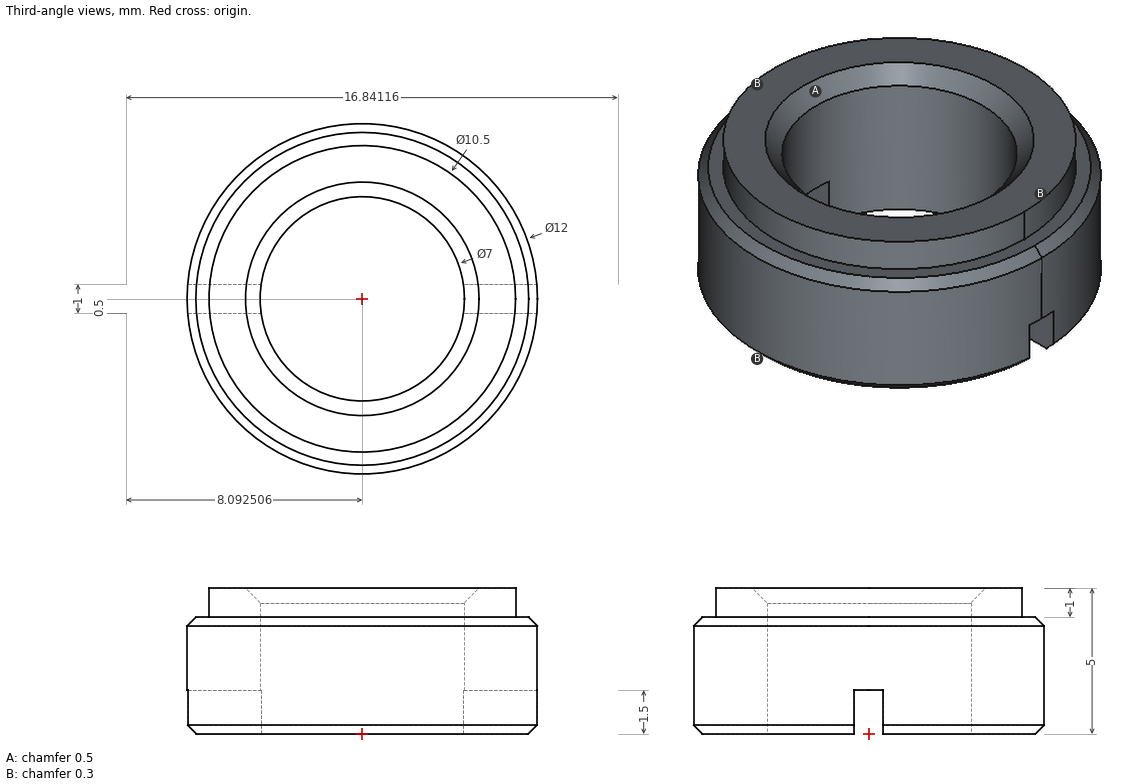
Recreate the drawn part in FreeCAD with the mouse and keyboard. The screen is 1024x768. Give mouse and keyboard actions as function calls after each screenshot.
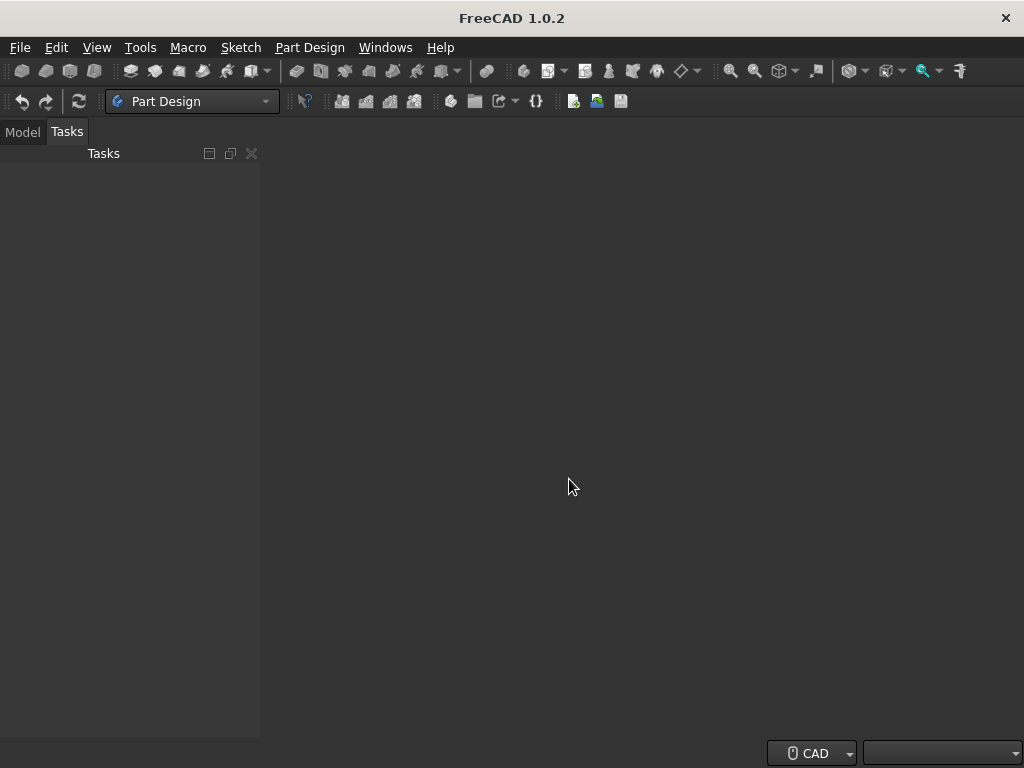
click(574, 102)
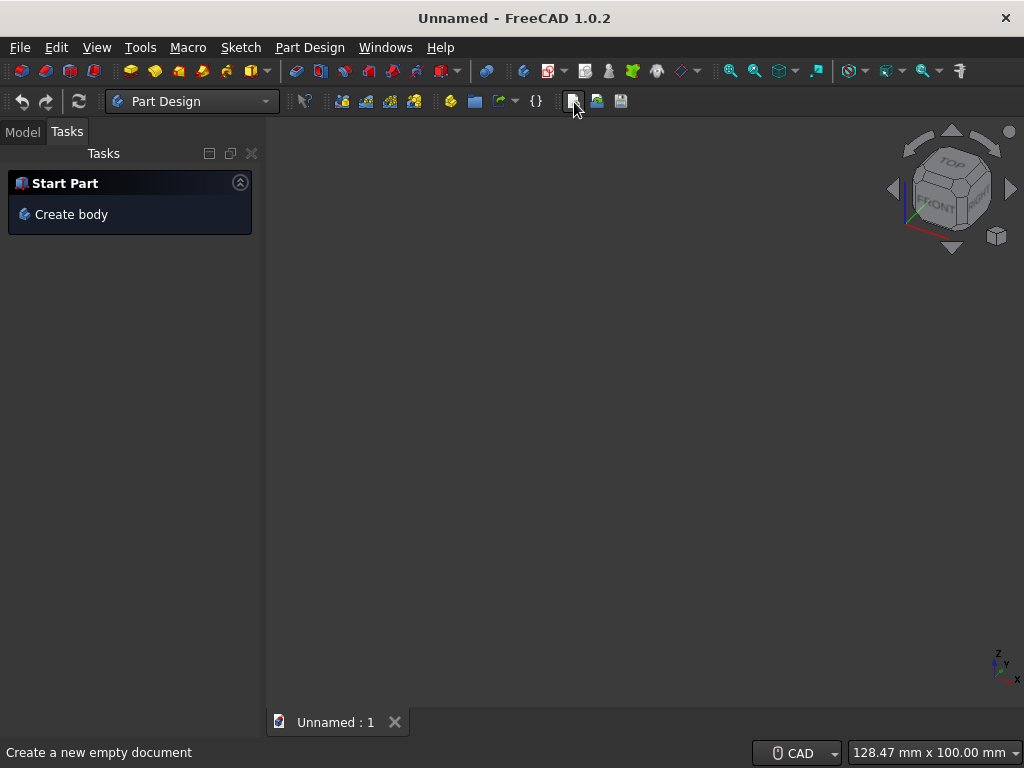
click(548, 72)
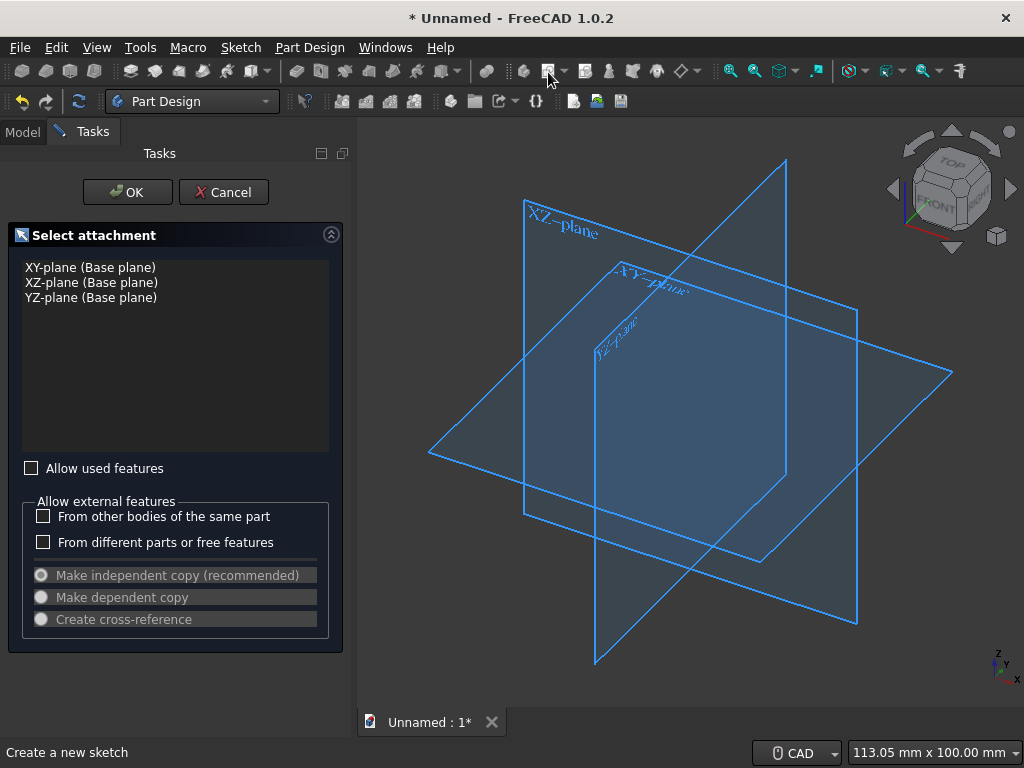
click(82, 268)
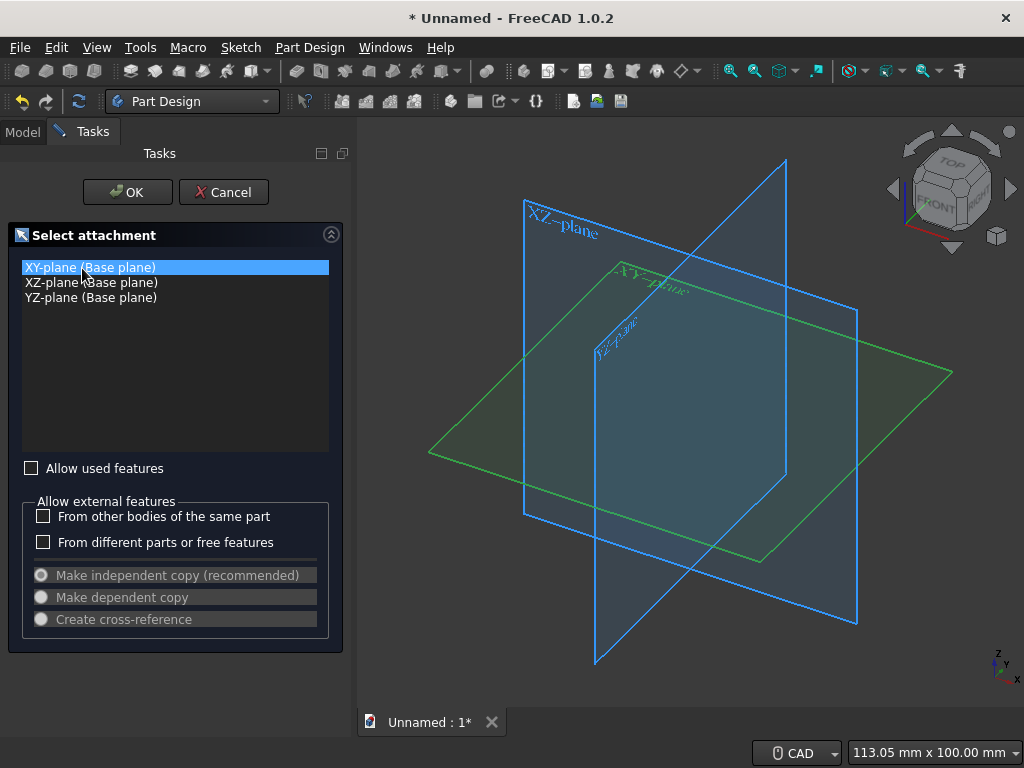
click(128, 192)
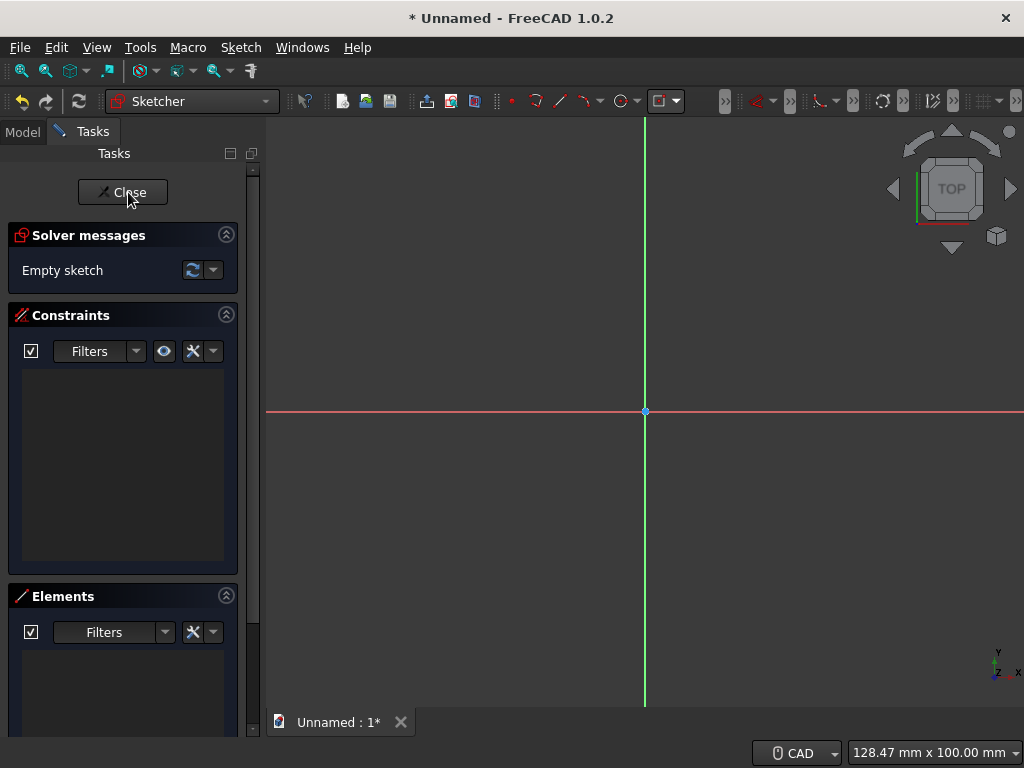
scroll(662, 412, up, 8)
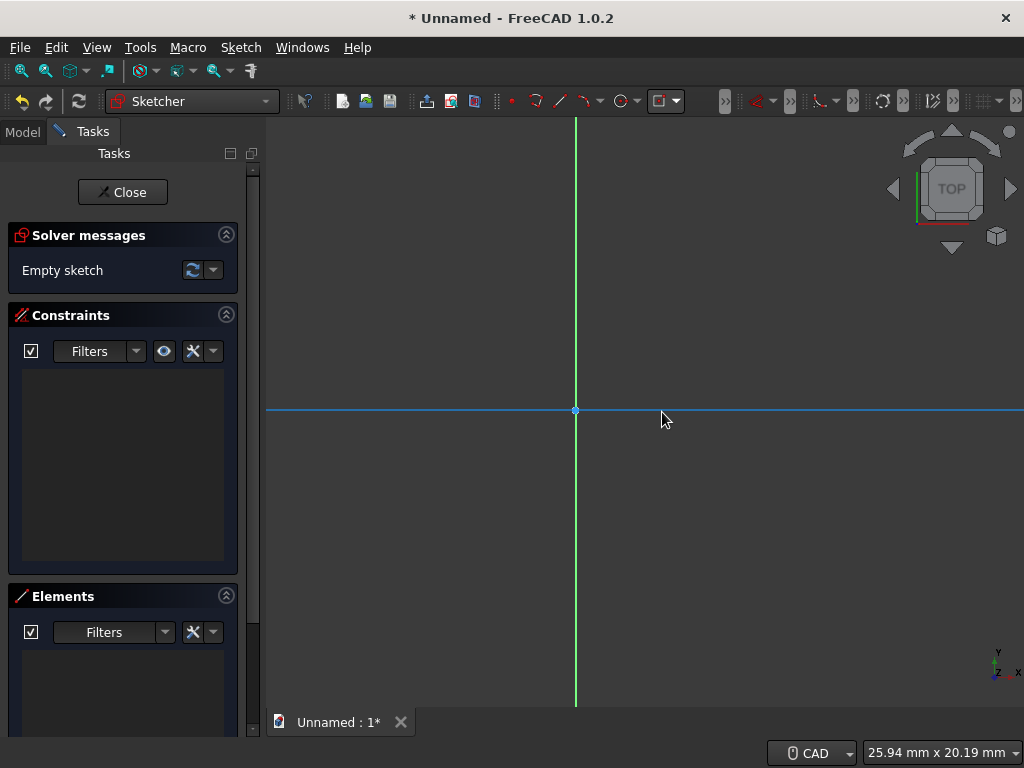
click(622, 102)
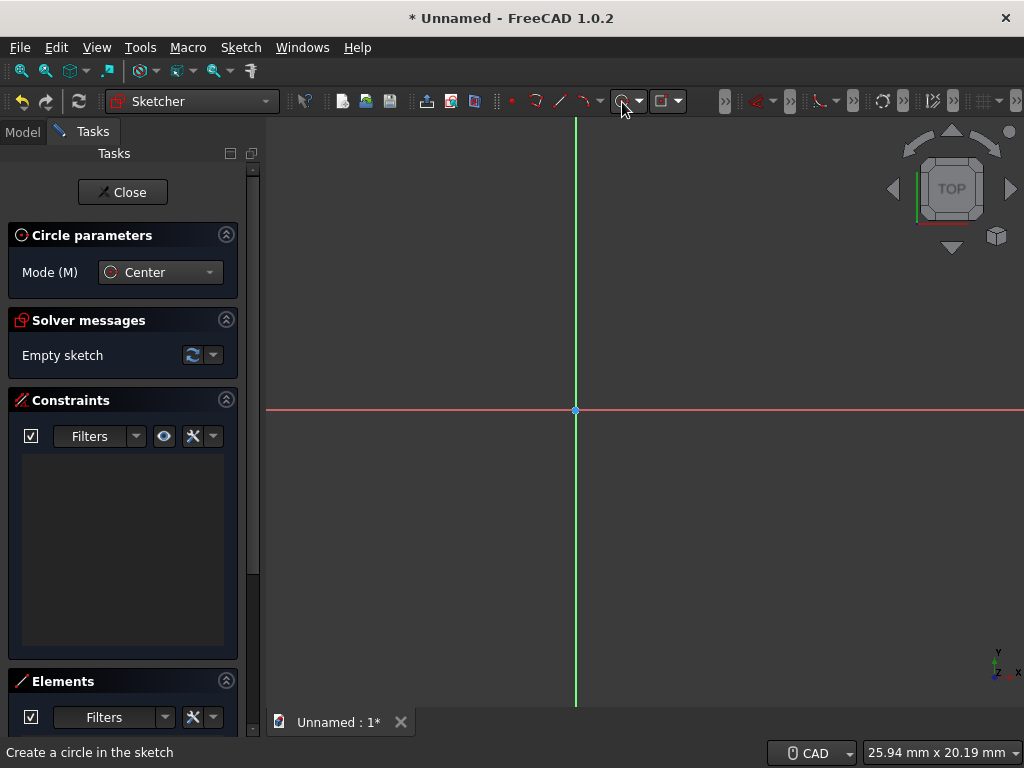
click(576, 410)
move(700, 286)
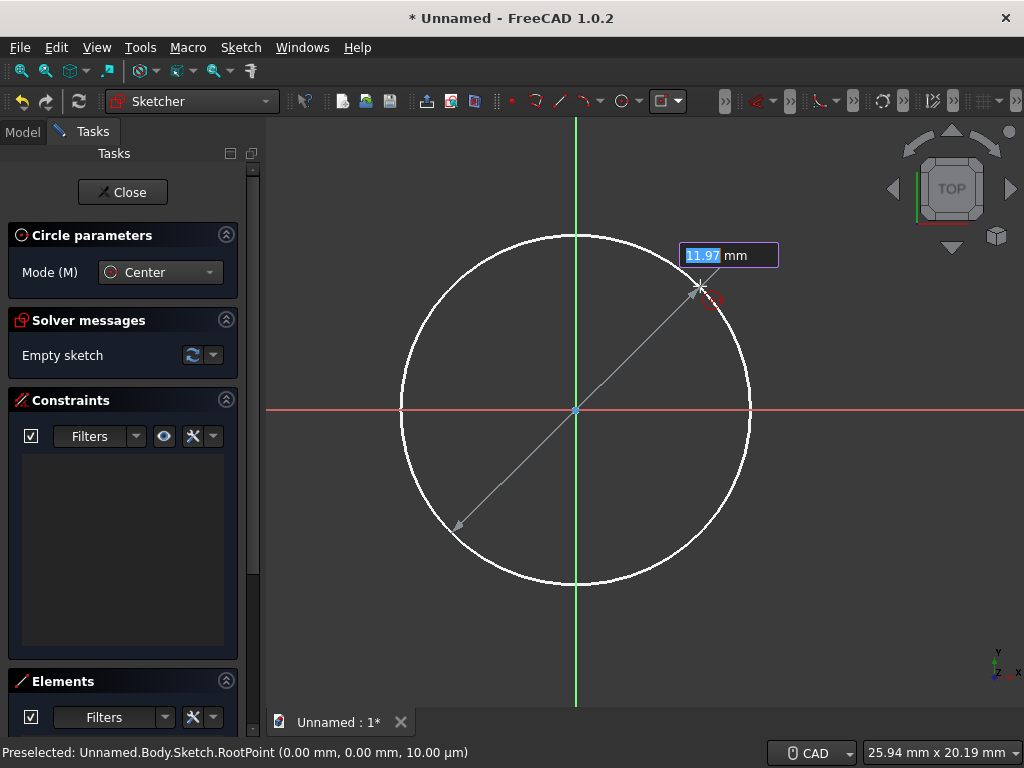
text(12)
key(Return)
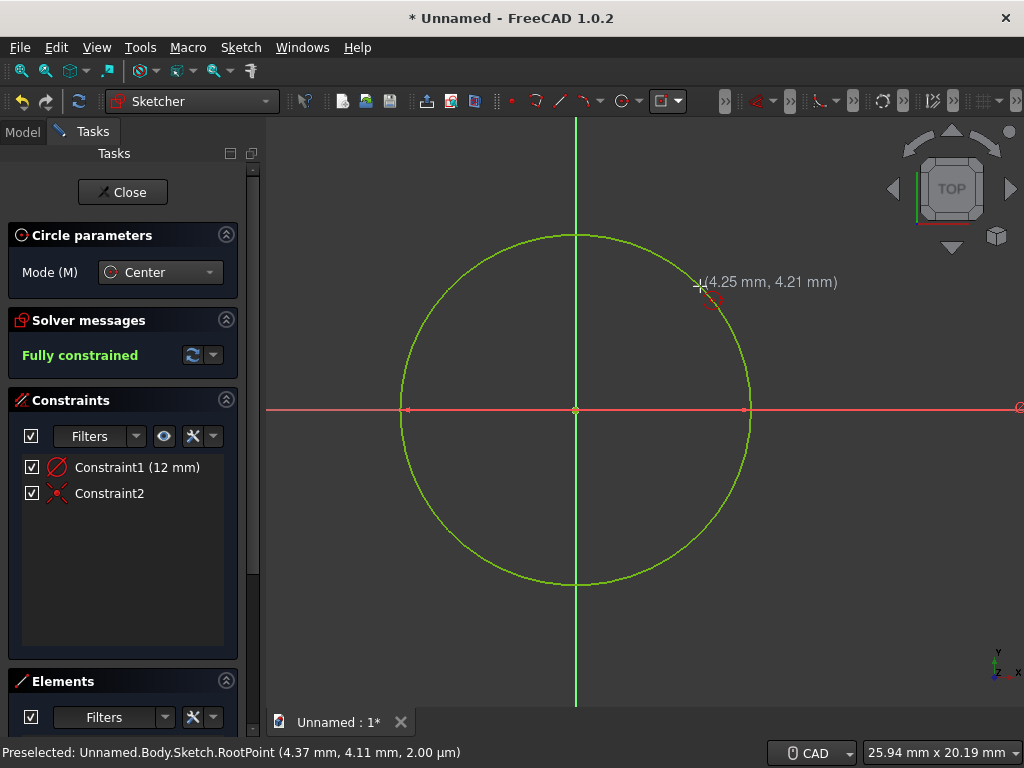
click(576, 410)
move(648, 338)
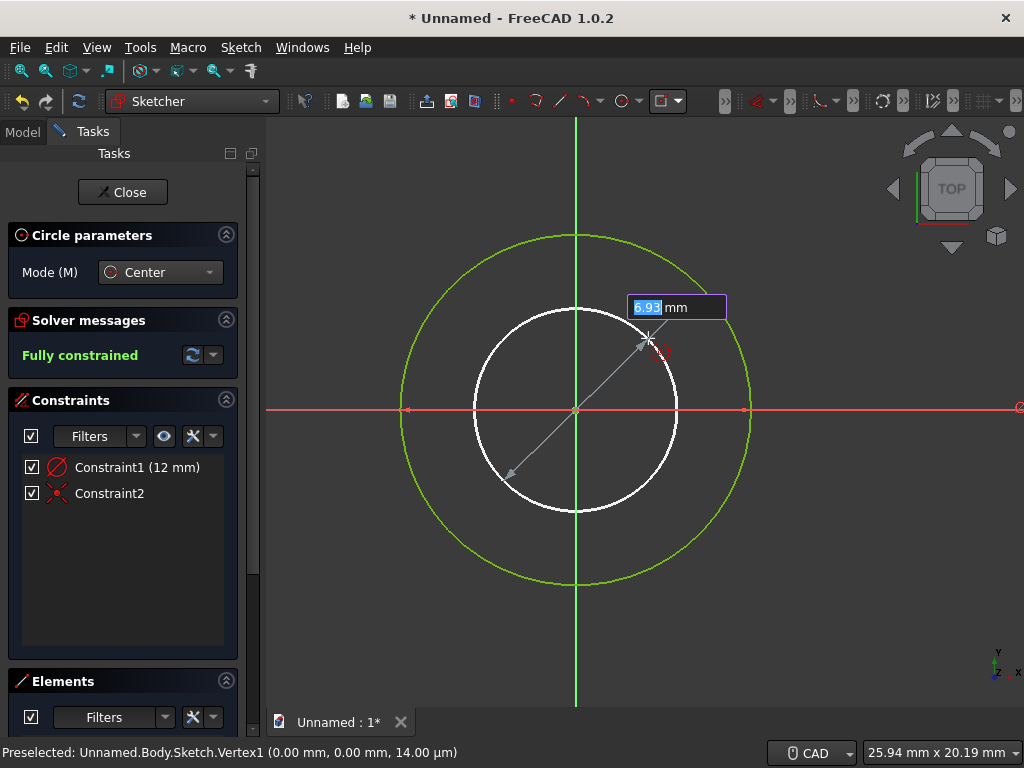
text(7)
key(Return)
key(Escape)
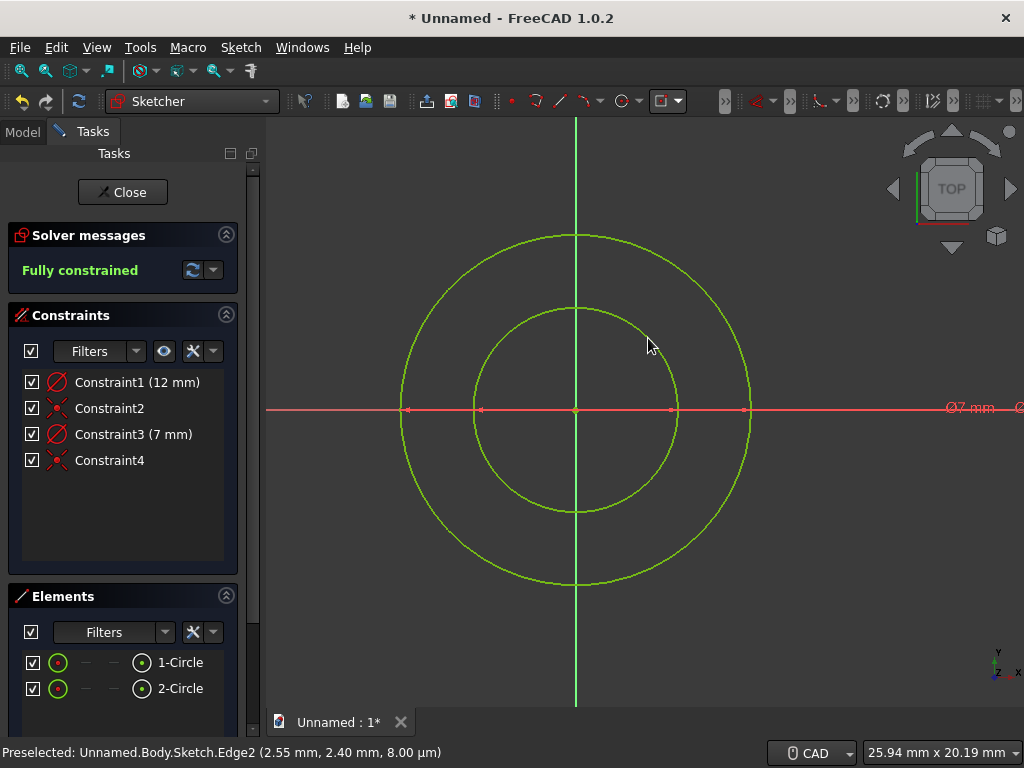
click(123, 192)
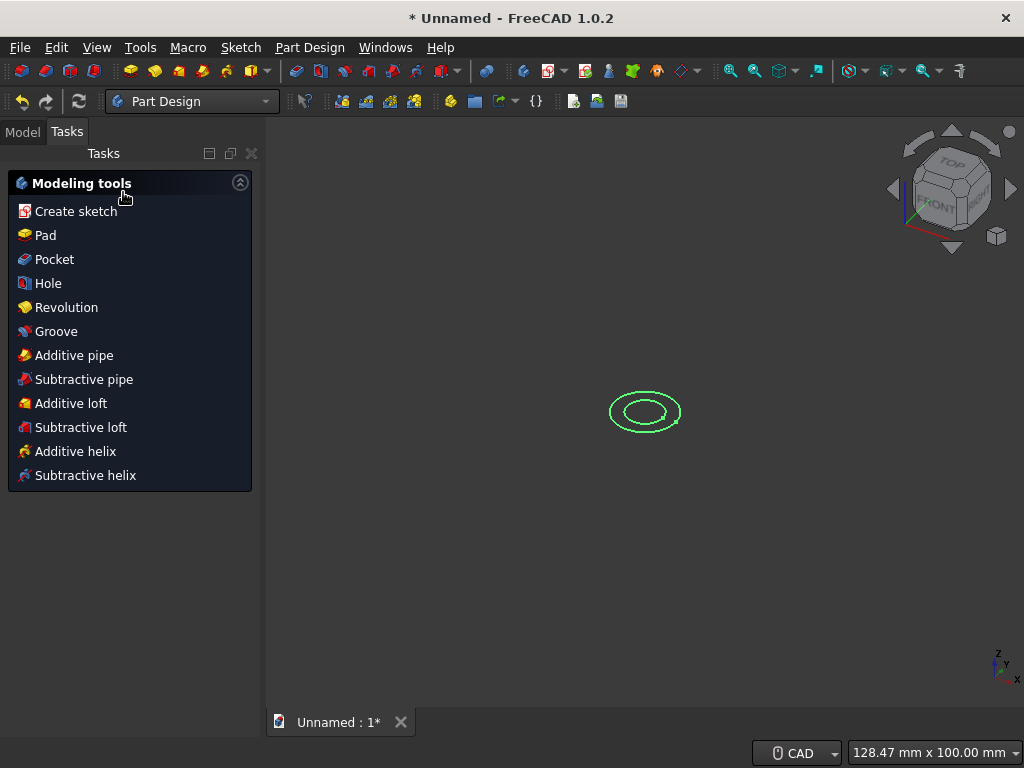
click(132, 72)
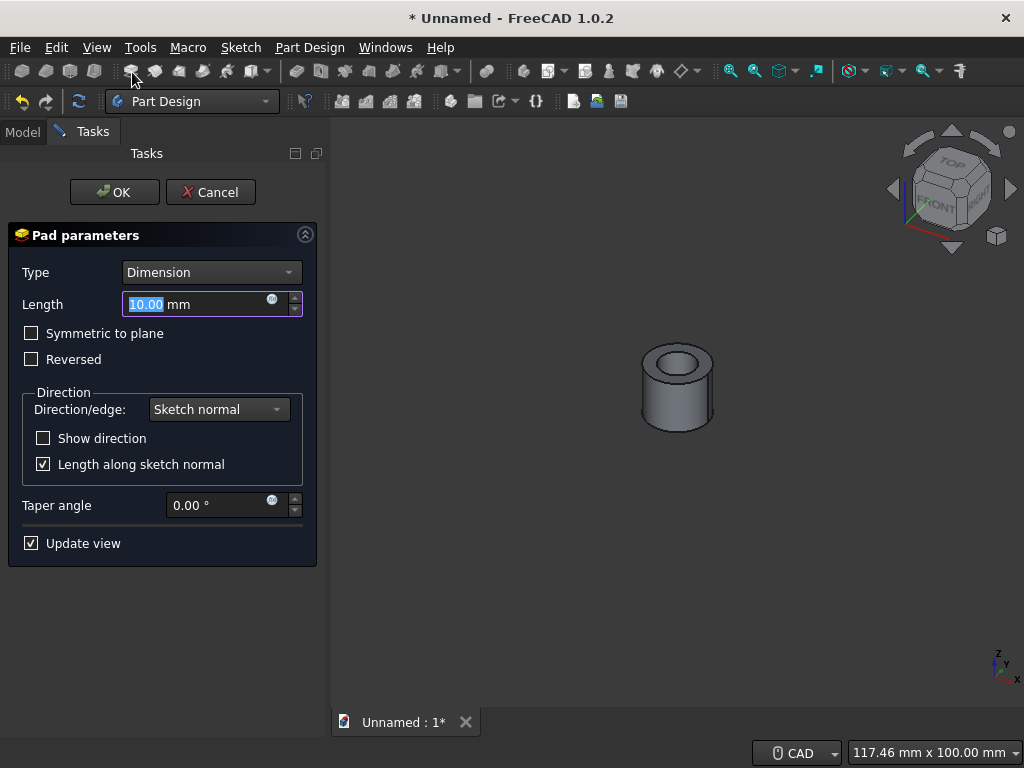
text(5)
key(Tab)